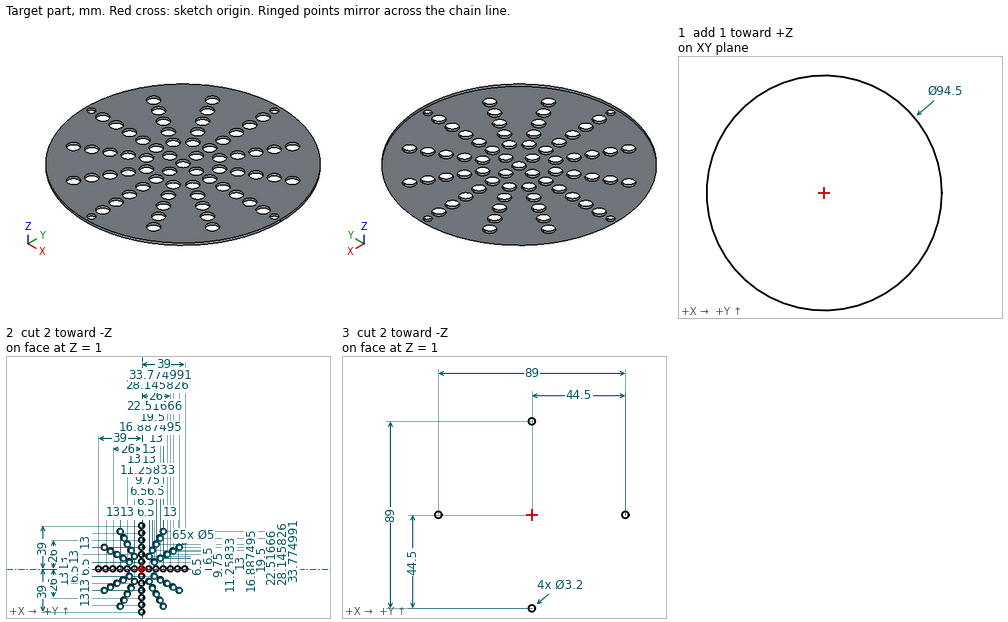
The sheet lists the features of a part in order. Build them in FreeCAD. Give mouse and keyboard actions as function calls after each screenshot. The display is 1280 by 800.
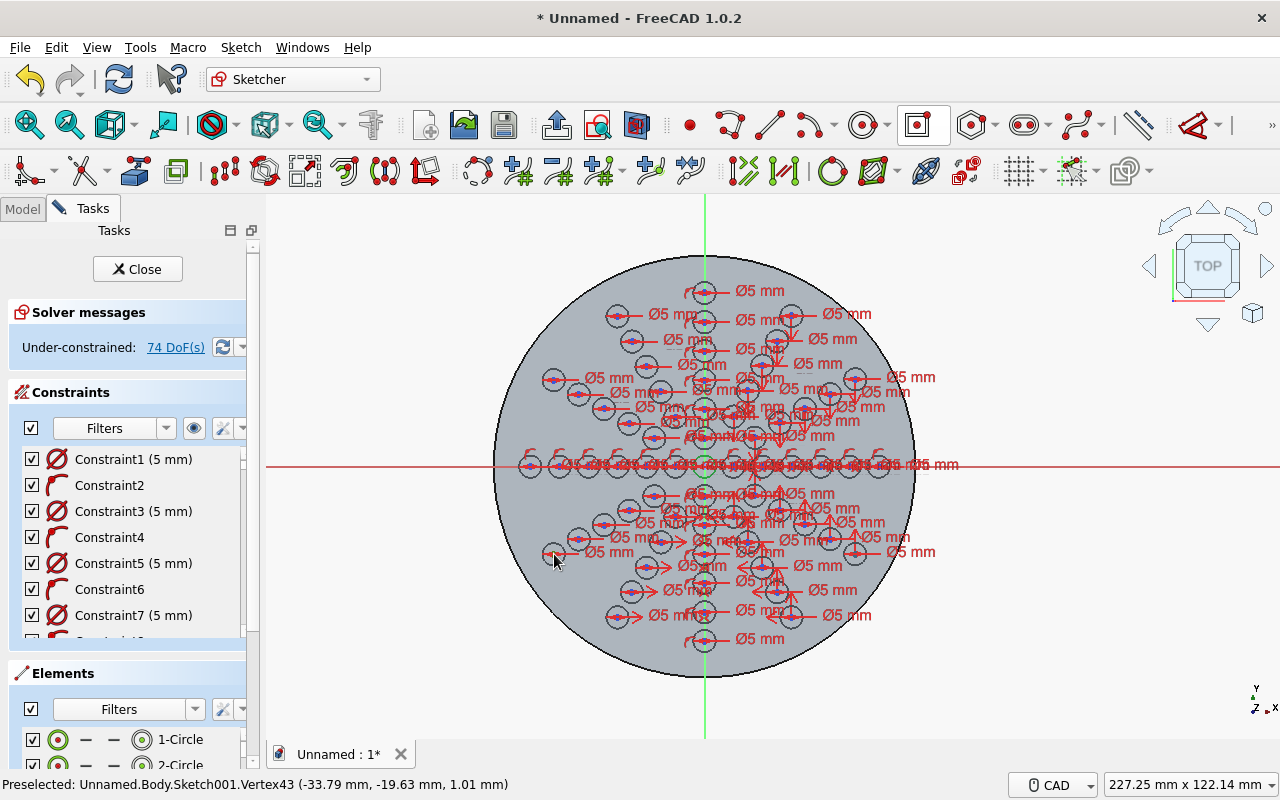
click(705, 257)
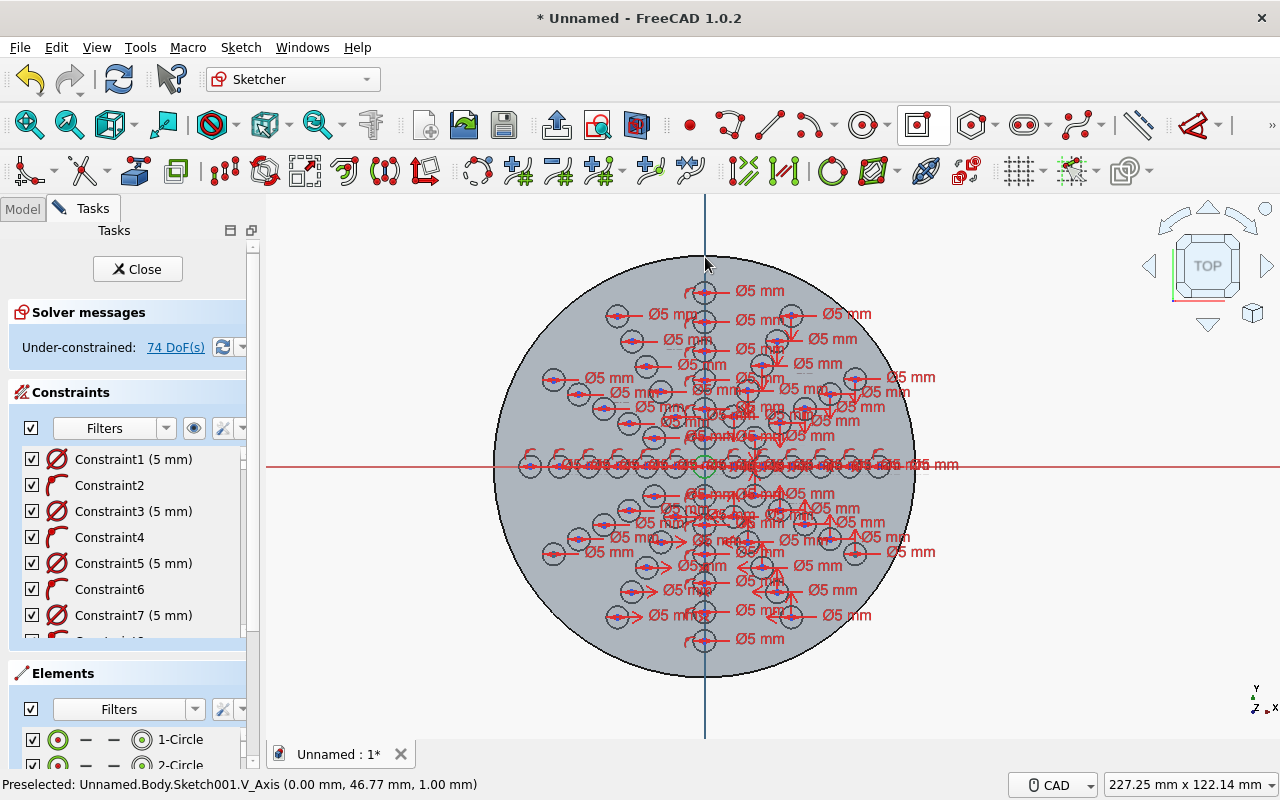
key(s)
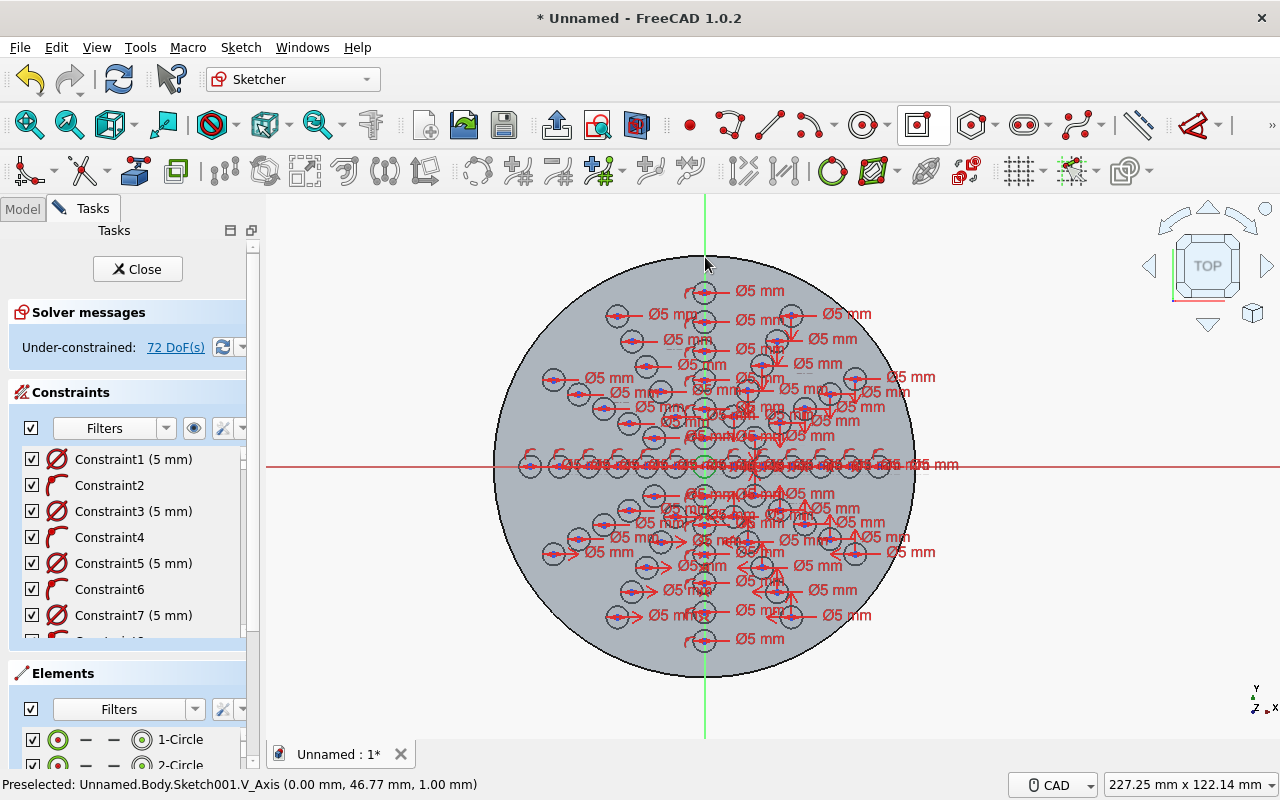
click(830, 539)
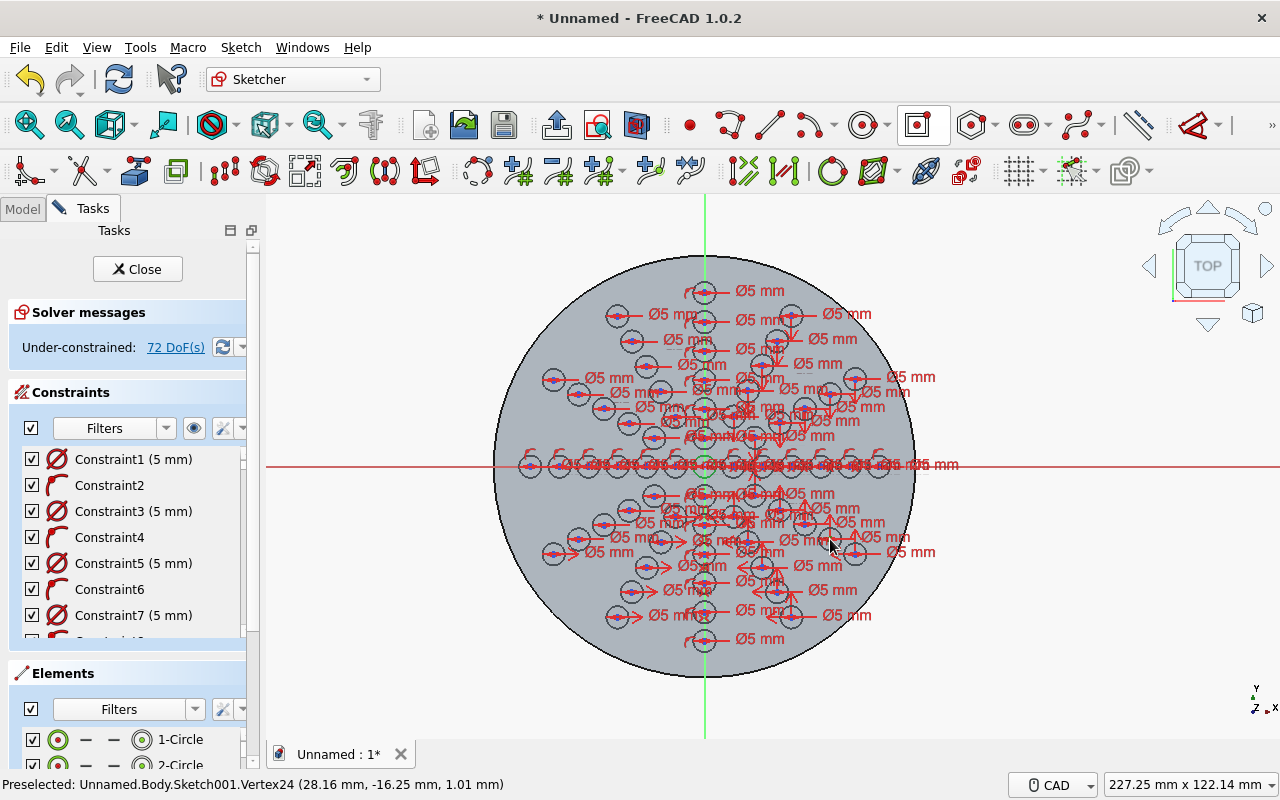
click(579, 539)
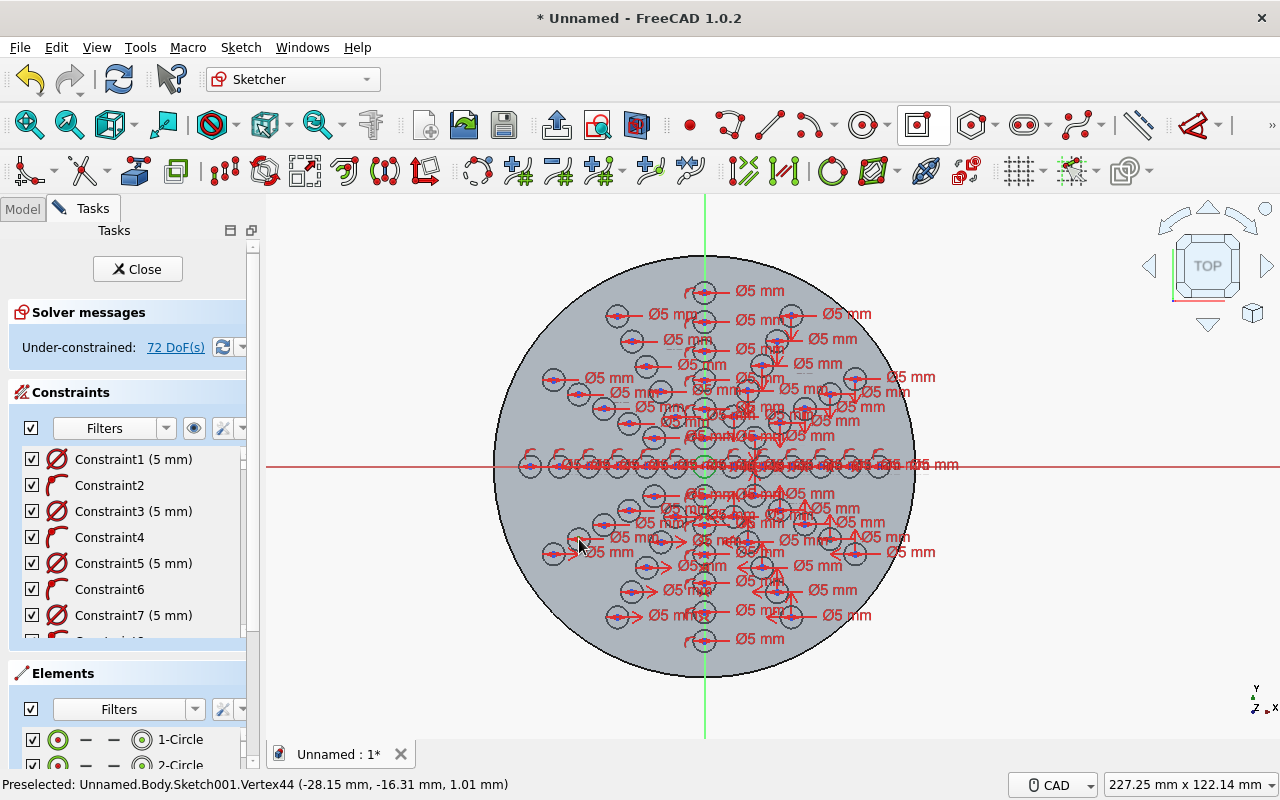
click(705, 257)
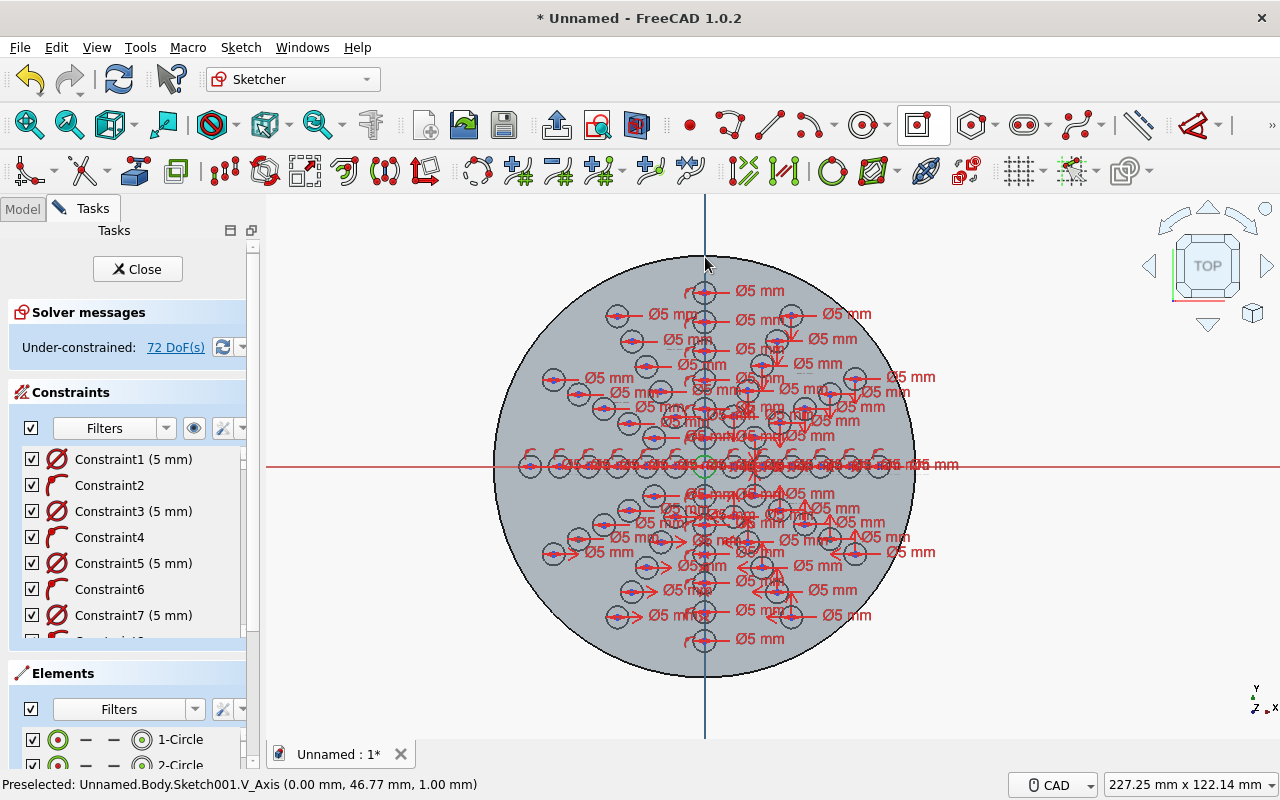
key(s)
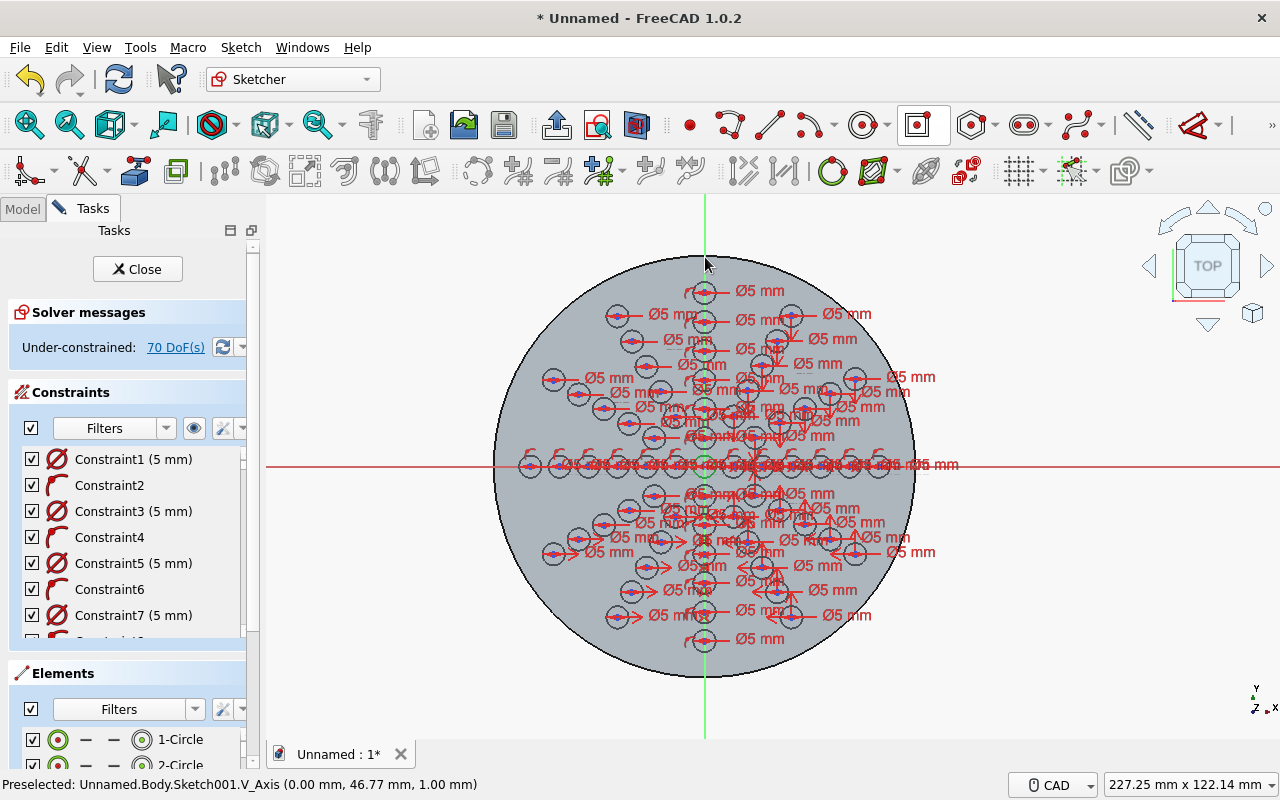
click(805, 524)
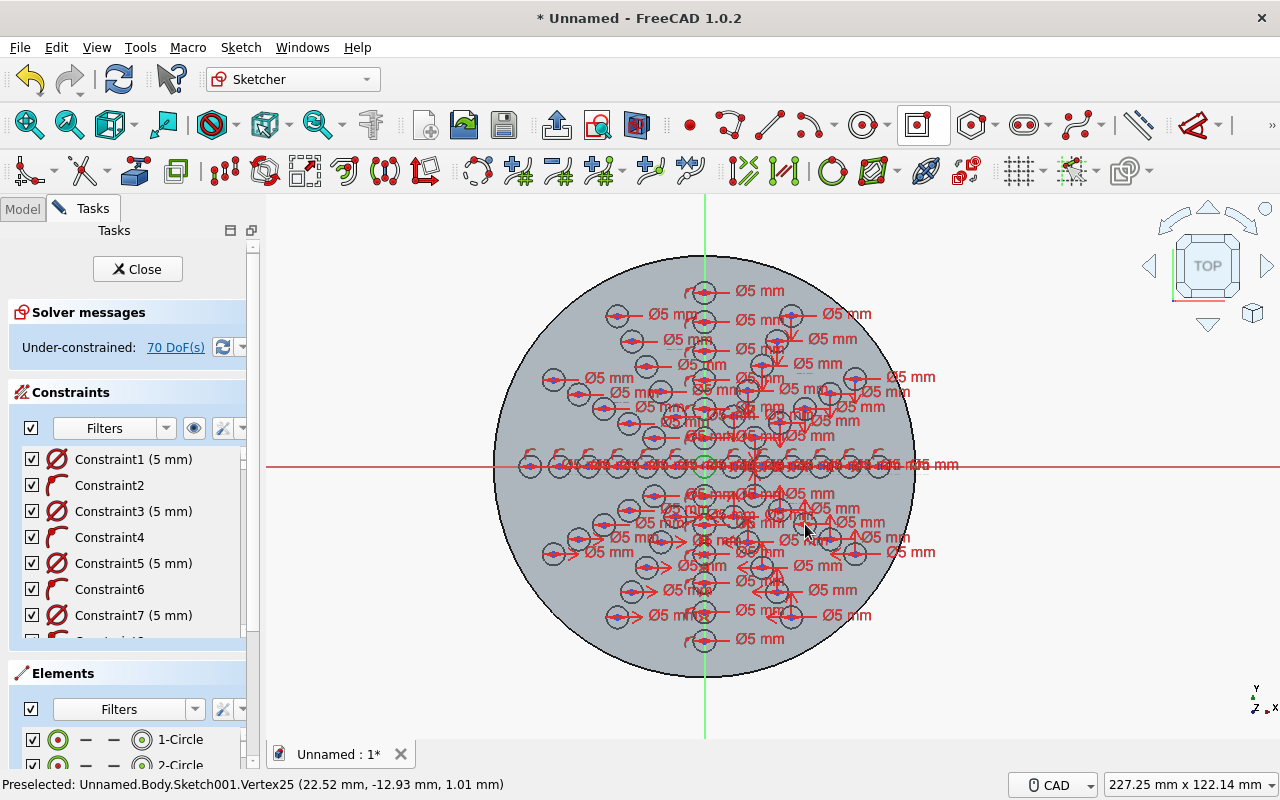
click(604, 525)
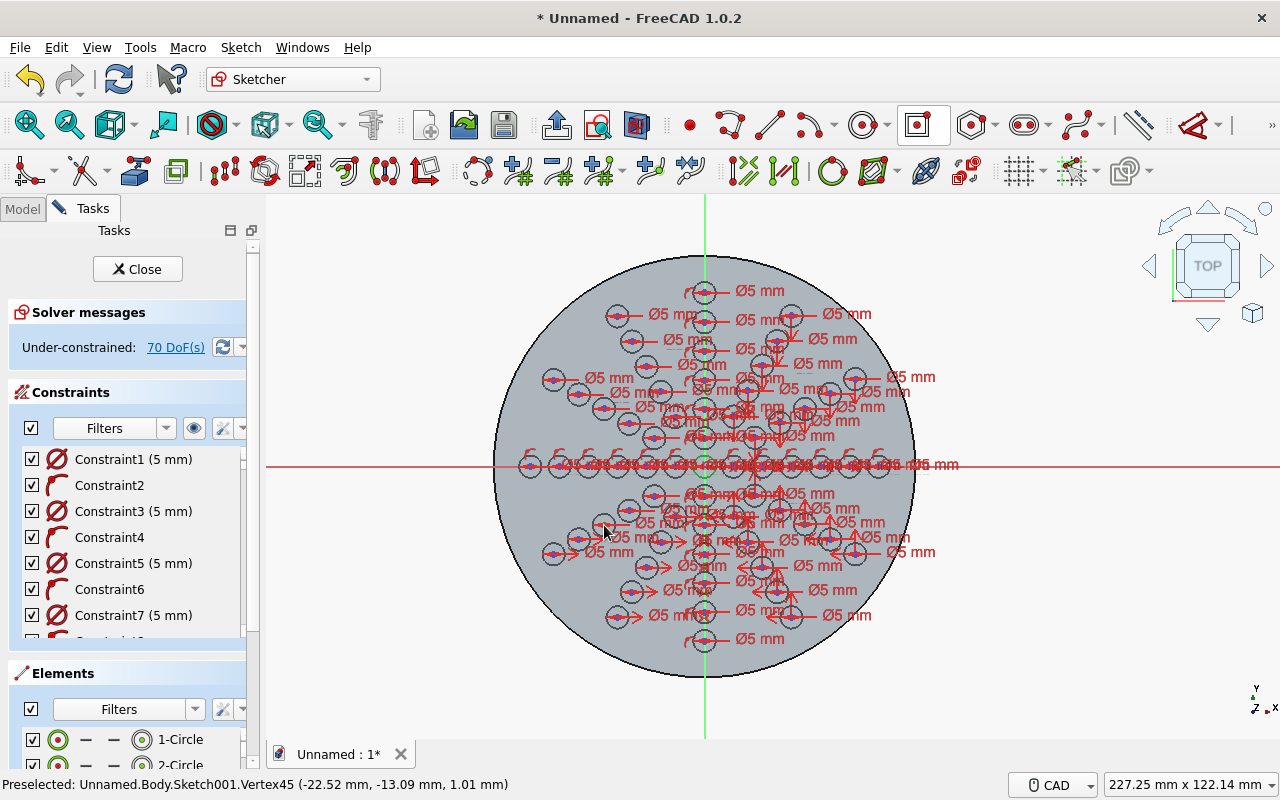
click(705, 257)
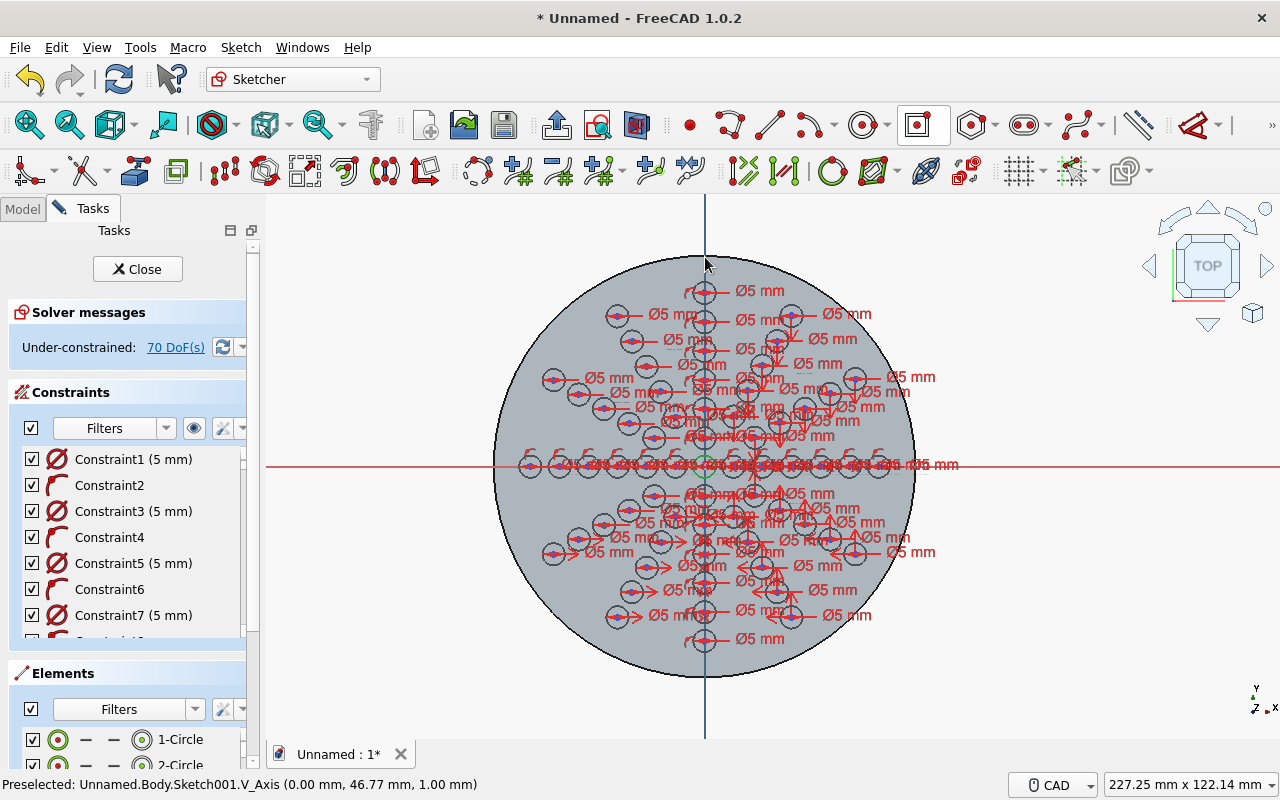
key(s)